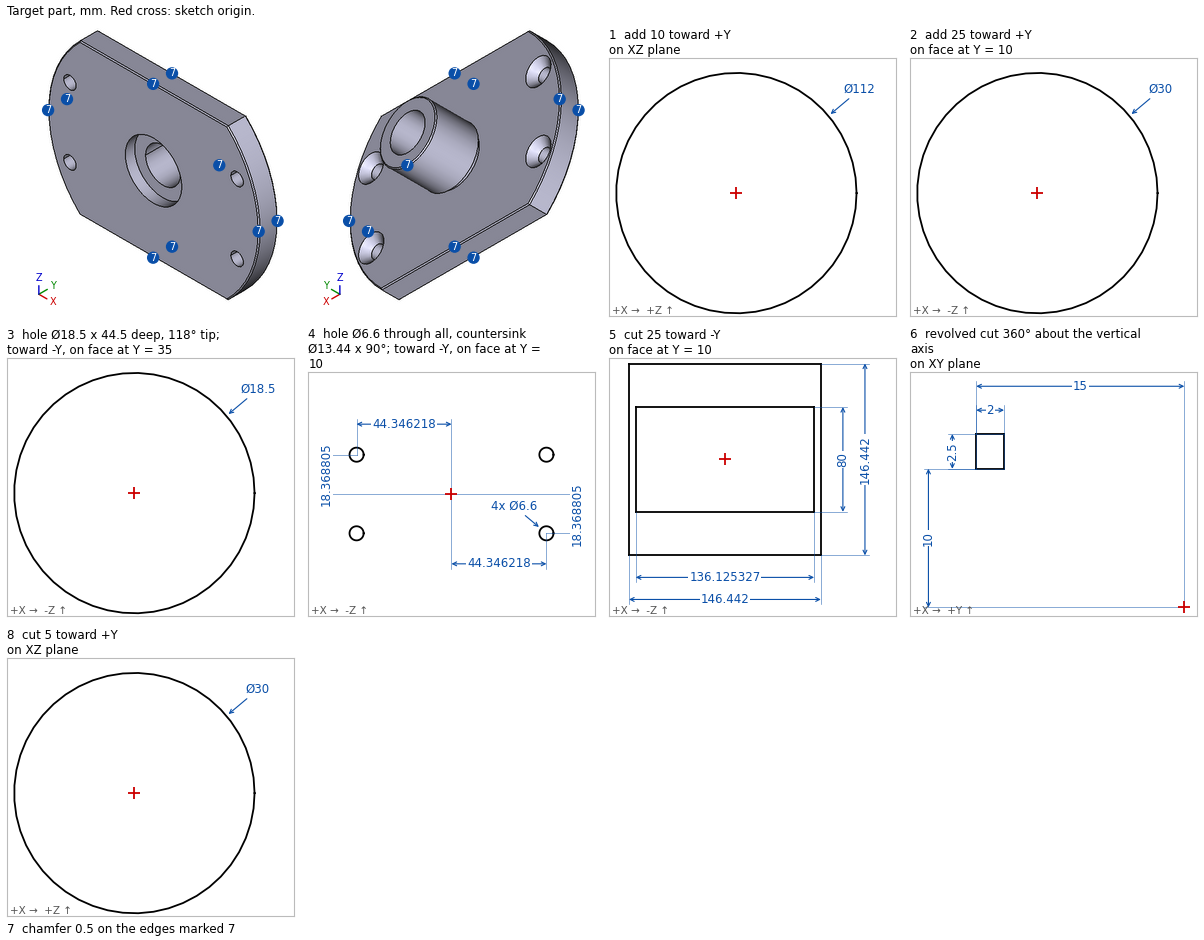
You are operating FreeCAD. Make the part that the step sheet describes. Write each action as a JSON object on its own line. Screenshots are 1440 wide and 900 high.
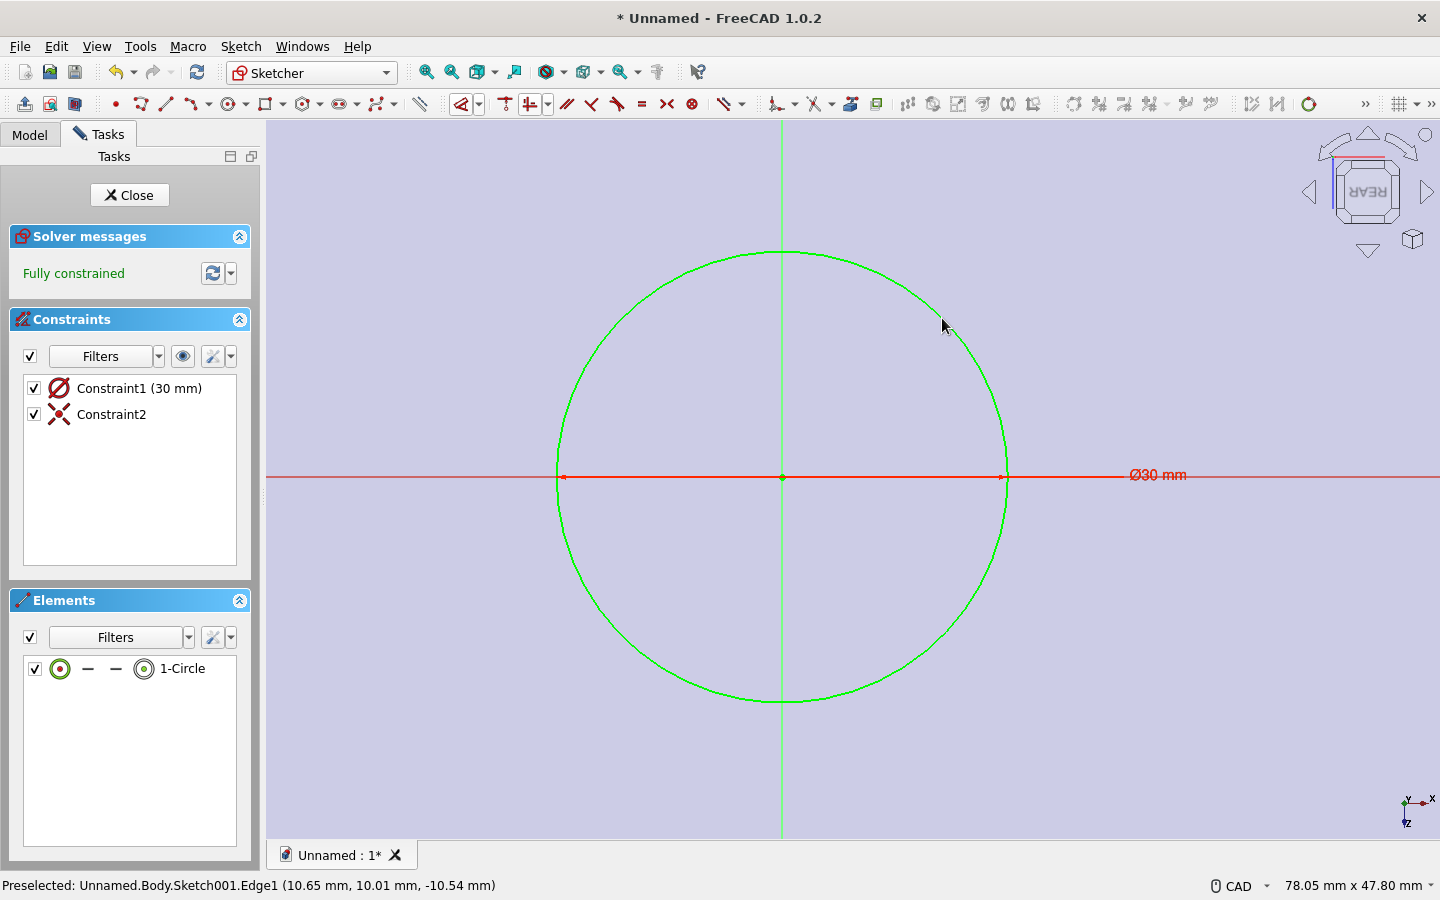
{"action": "left_click", "coordinate": [130, 195]}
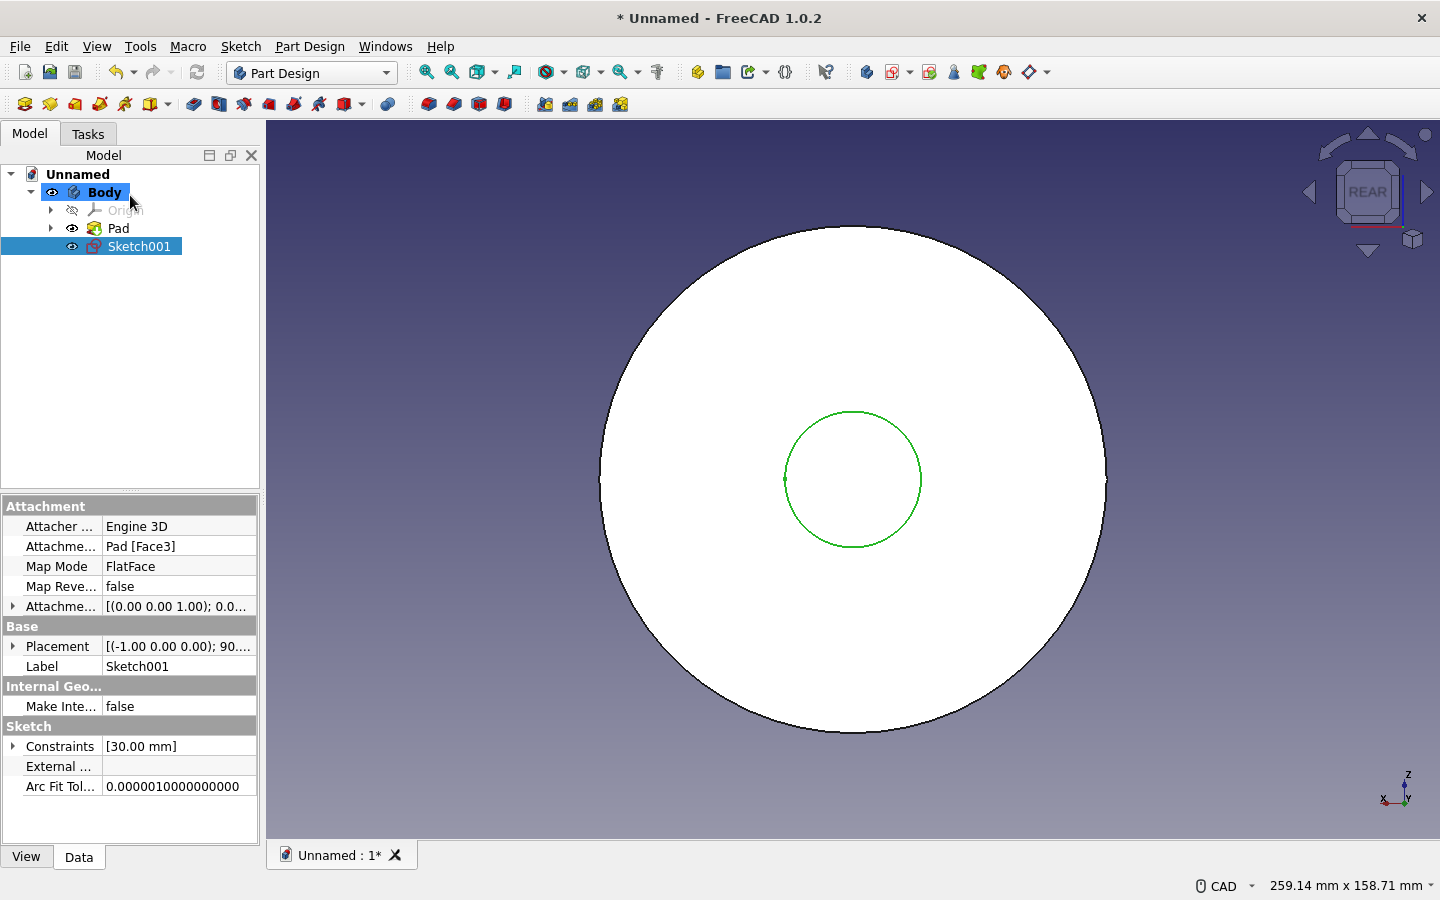
{"action": "left_click", "coordinate": [25, 104]}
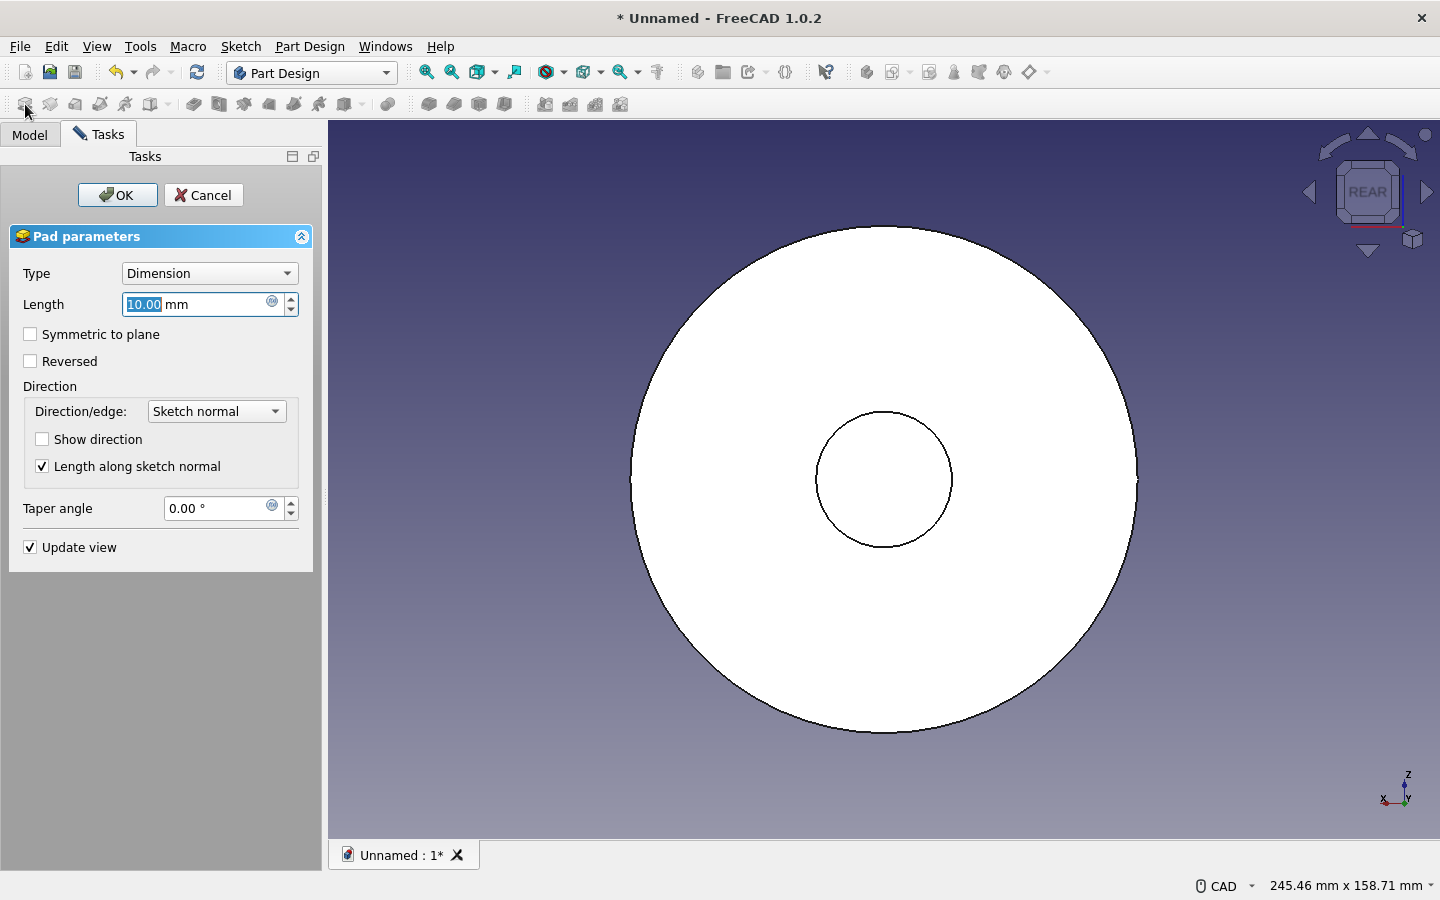
{"action": "type", "text": "25"}
{"action": "key", "text": "Tab"}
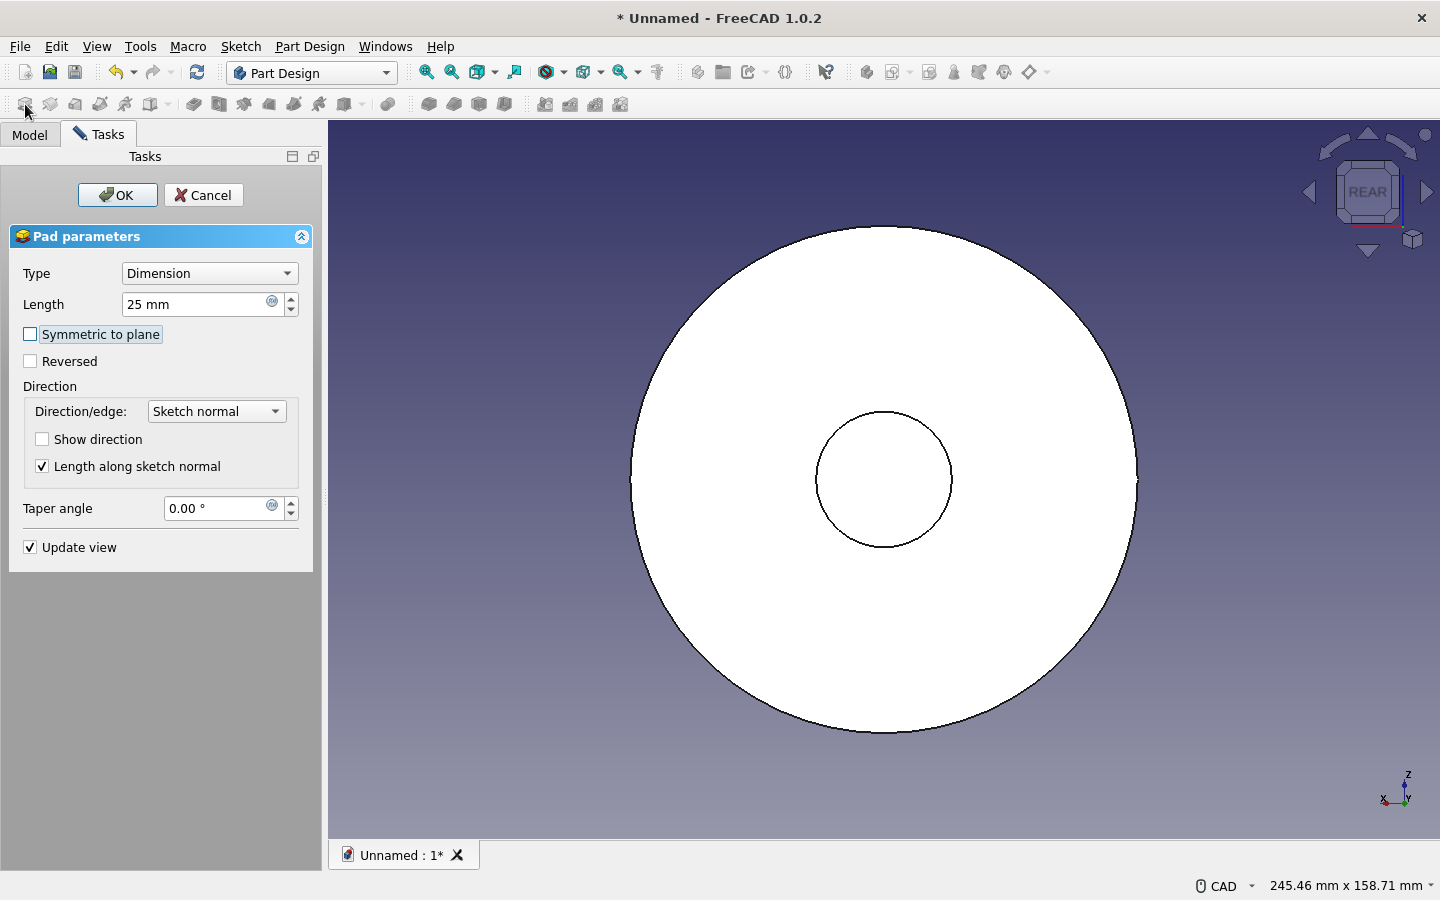
{"action": "left_click", "coordinate": [118, 195]}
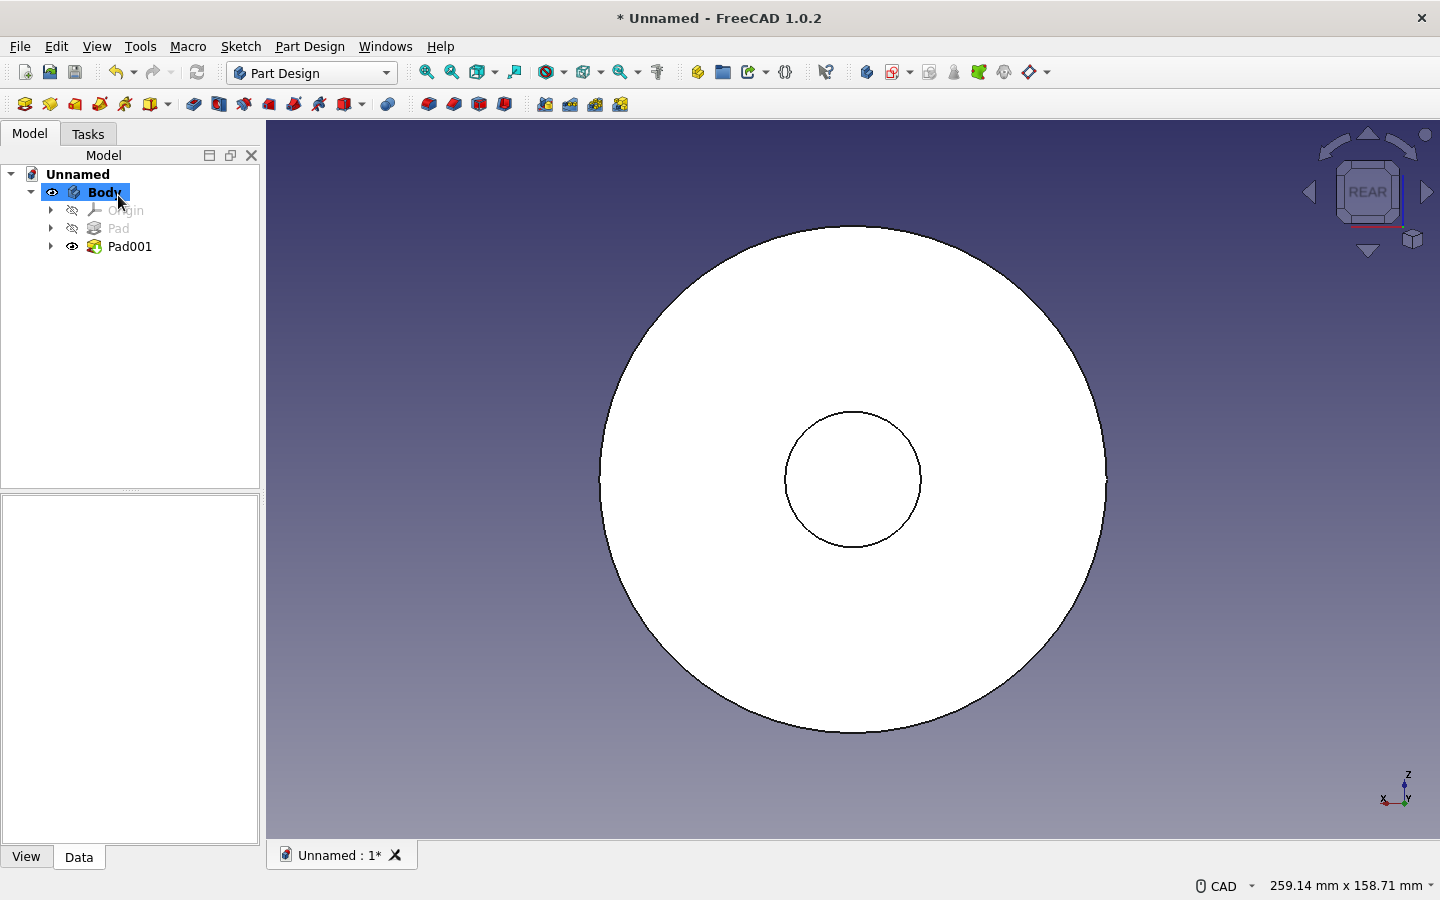
{"action": "left_click", "coordinate": [853, 478]}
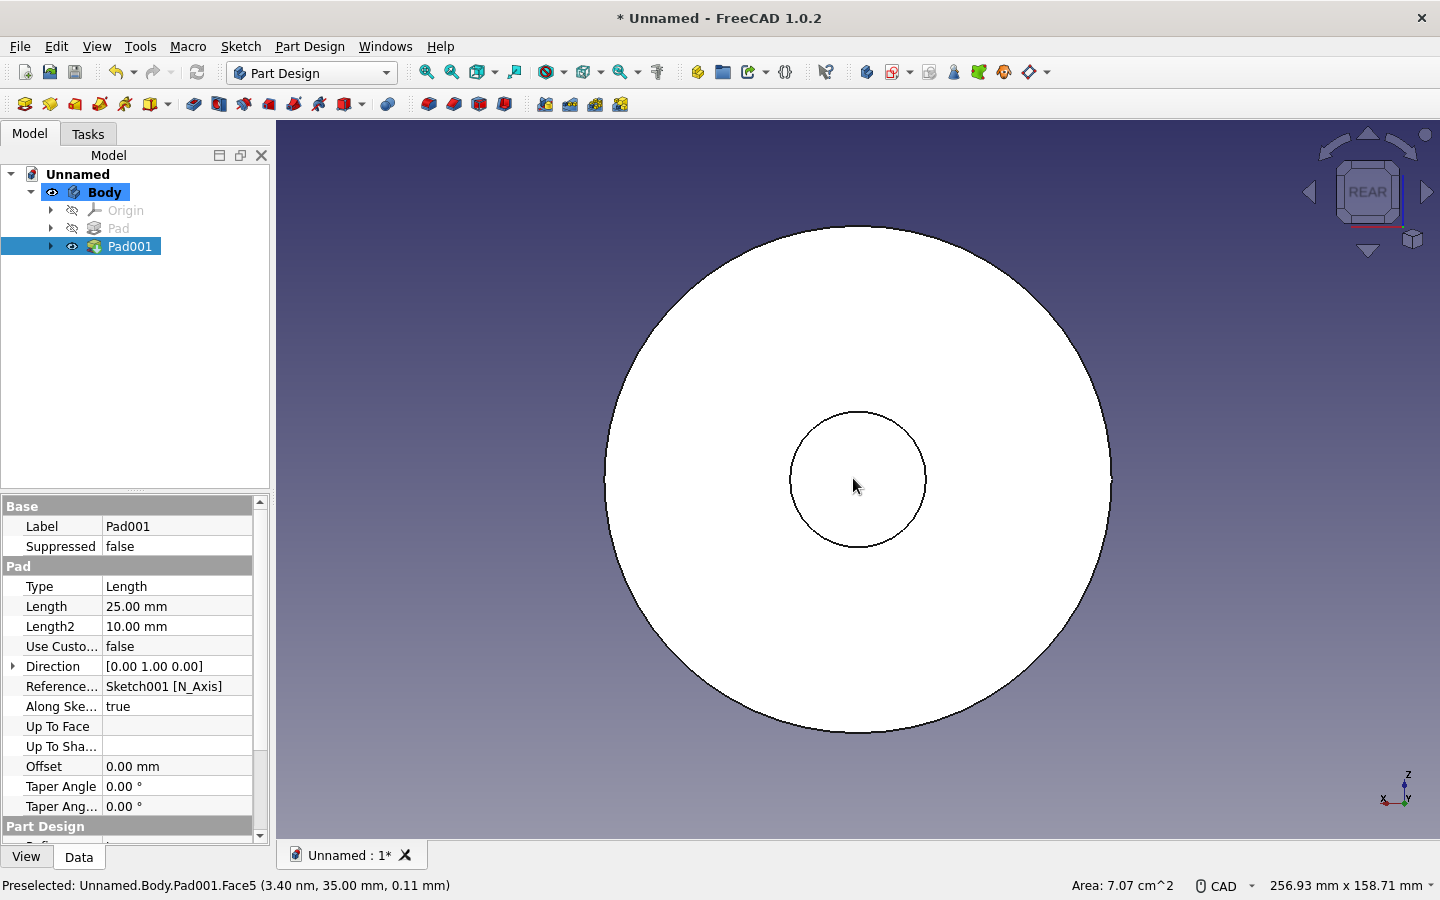
{"action": "left_click", "coordinate": [892, 72]}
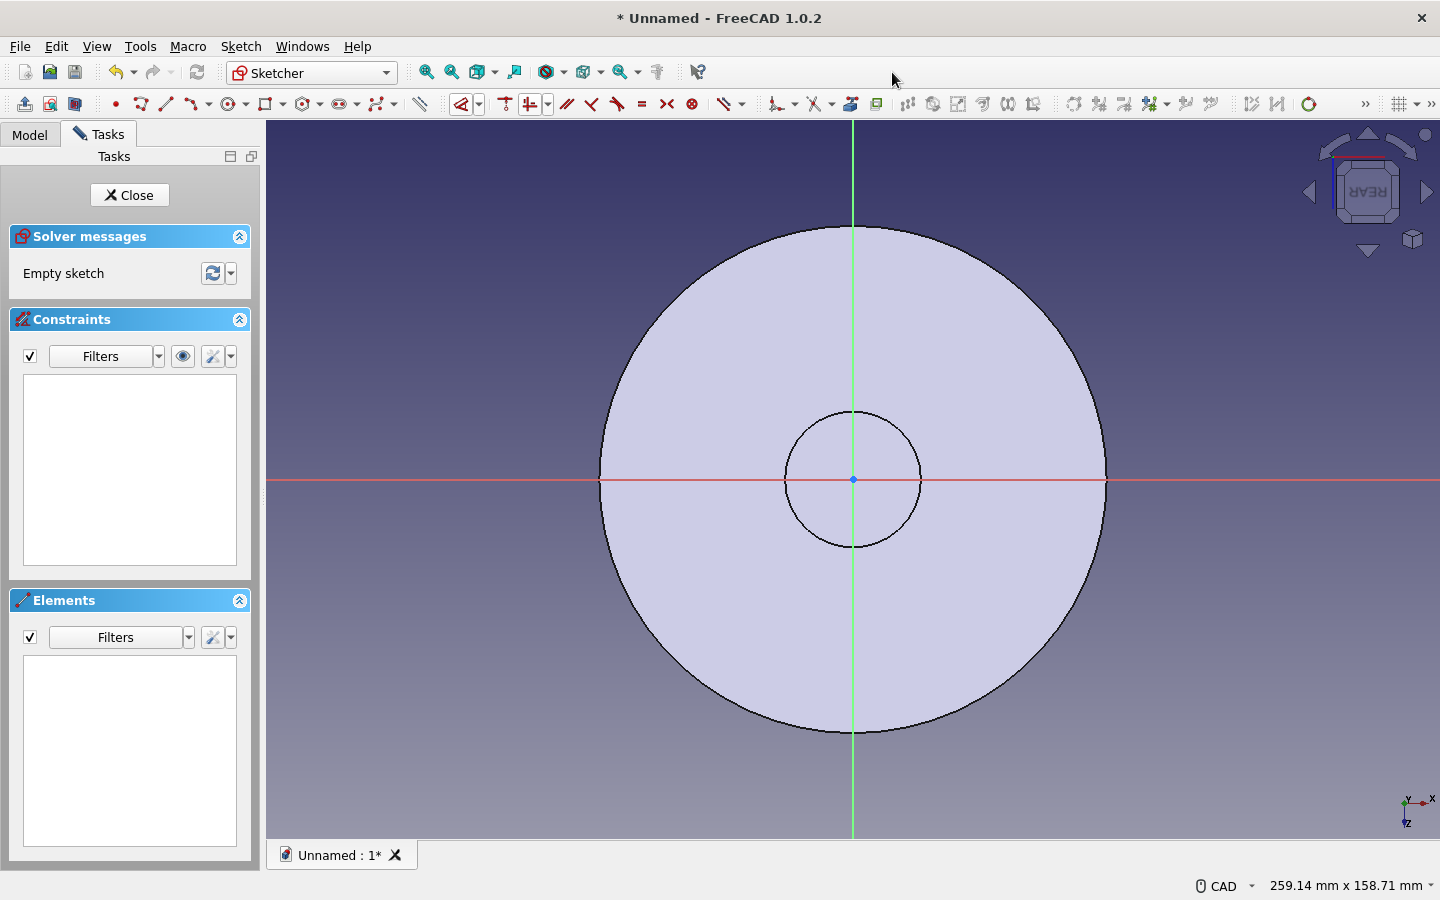
{"action": "scroll", "coordinate": [867, 479], "scroll_direction": "up", "scroll_amount": 9}